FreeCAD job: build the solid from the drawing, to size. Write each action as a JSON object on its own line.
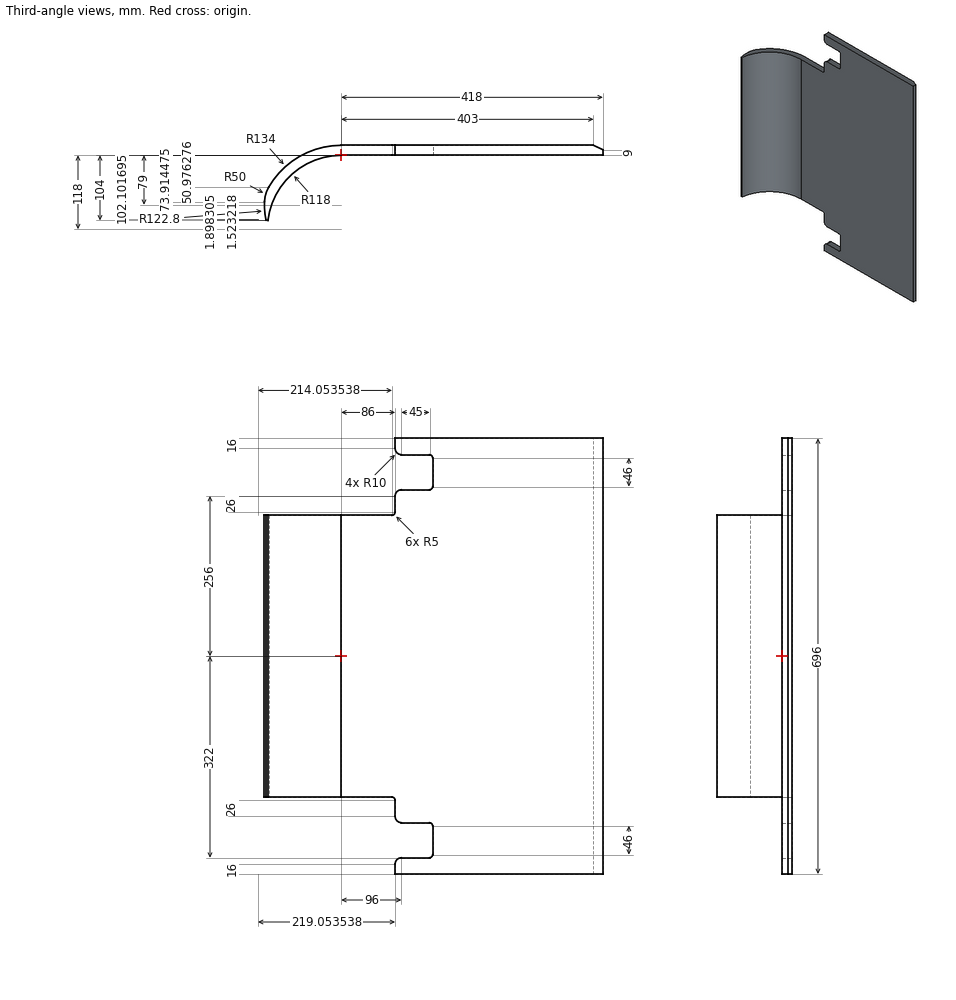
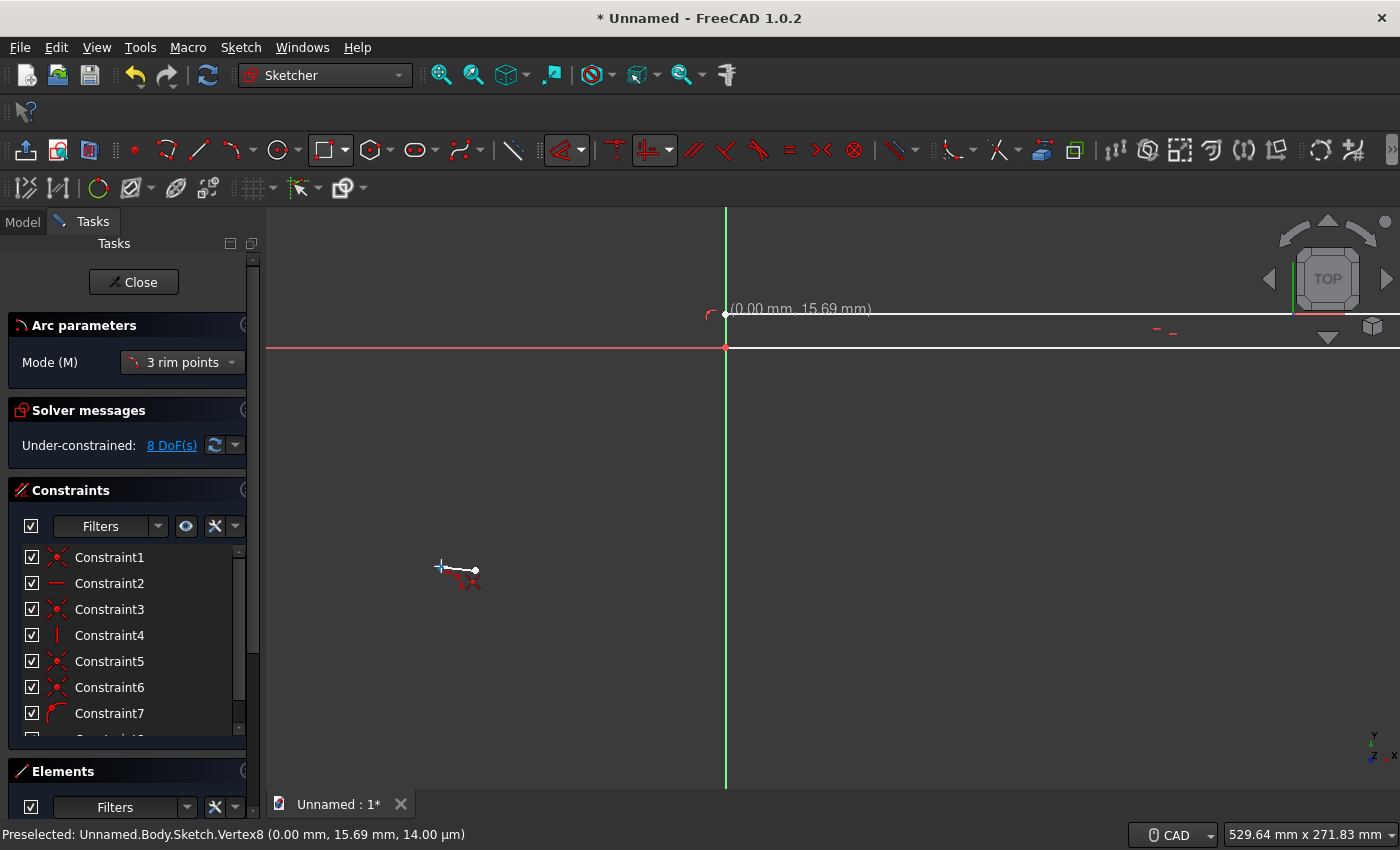
{"action": "left_click", "coordinate": [441, 567]}
{"action": "left_click", "coordinate": [535, 386]}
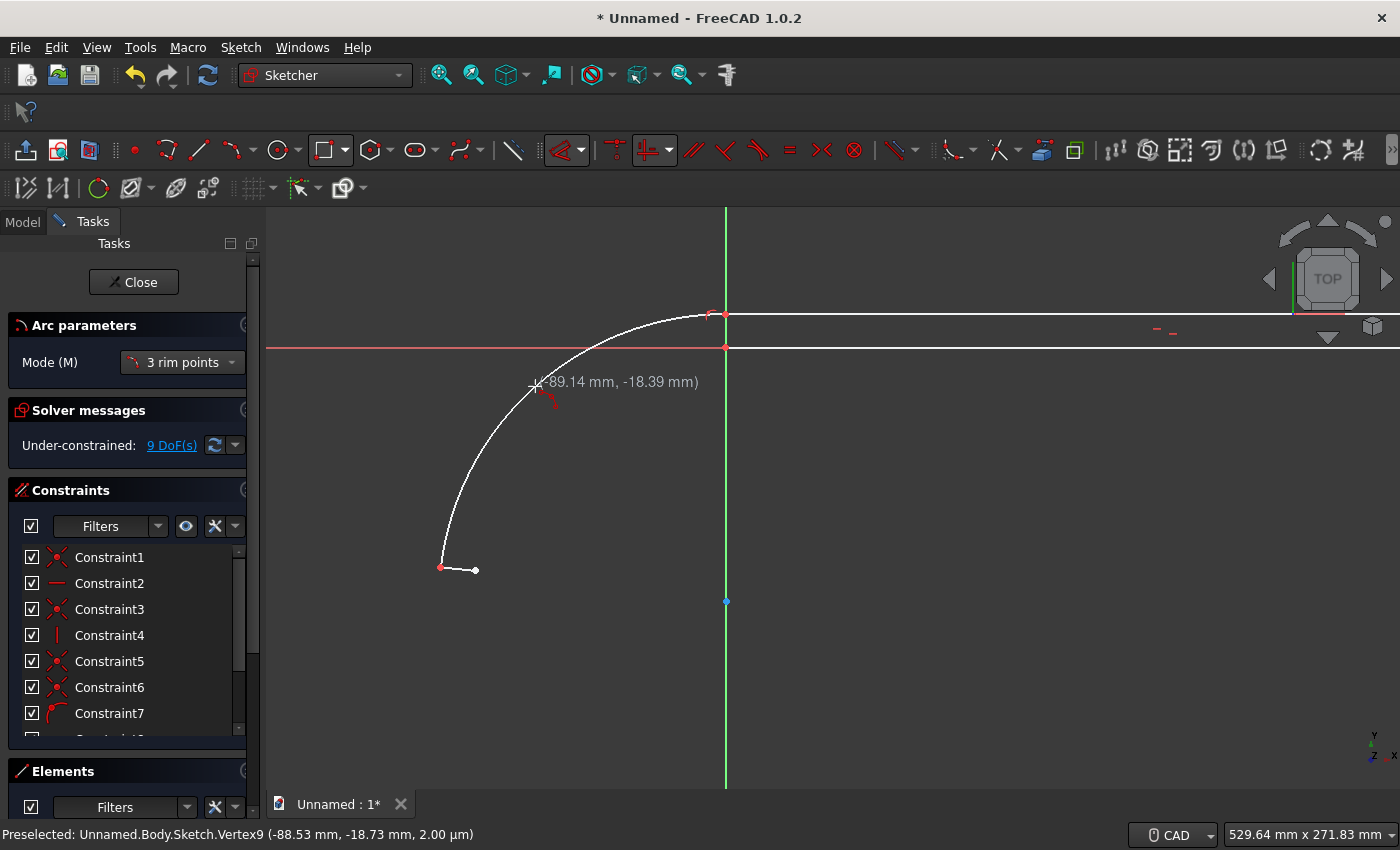
{"action": "left_click", "coordinate": [475, 571]}
{"action": "left_click", "coordinate": [726, 348]}
{"action": "left_click", "coordinate": [558, 411]}
{"action": "key", "text": "Escape"}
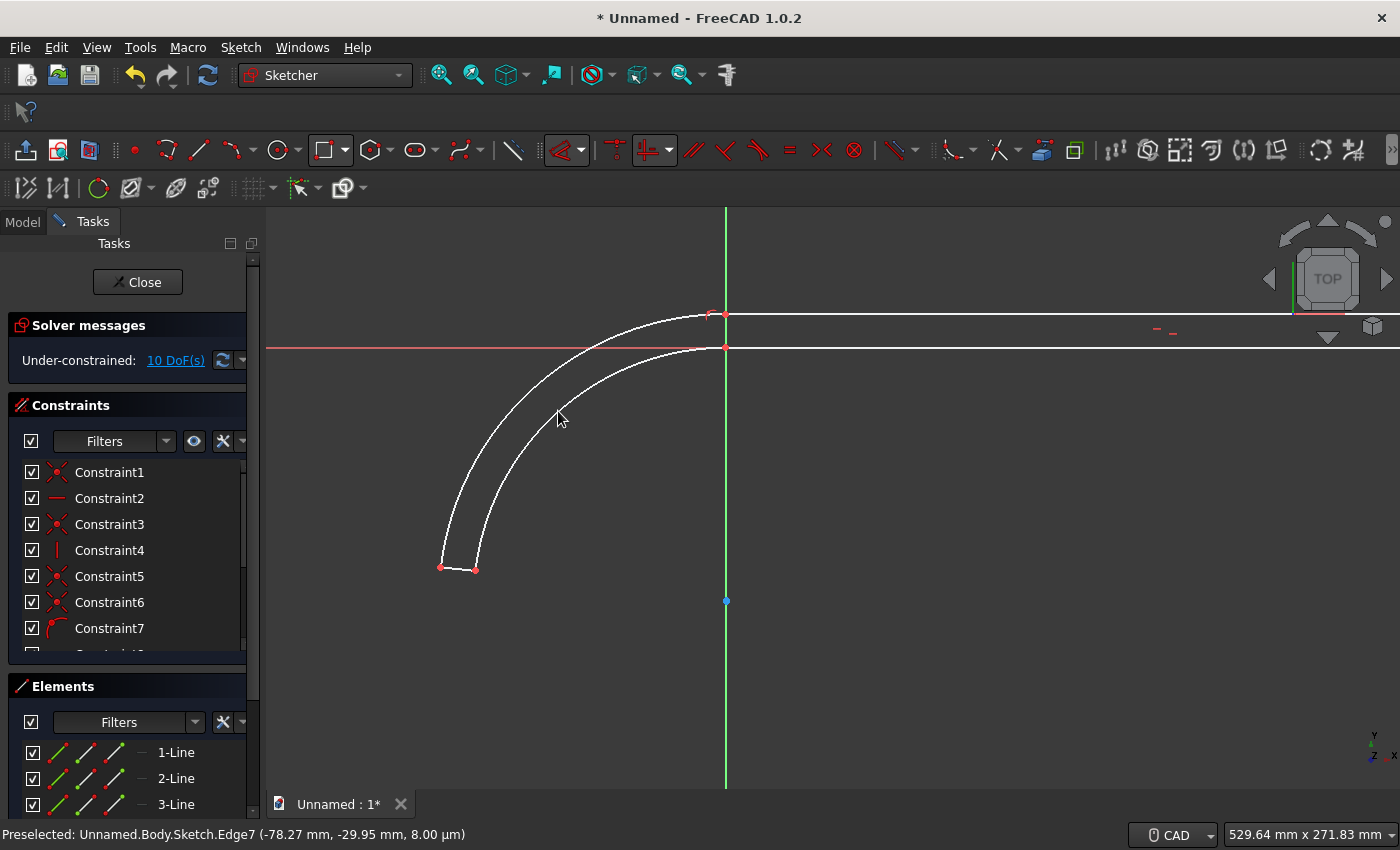
{"action": "left_click", "coordinate": [482, 450]}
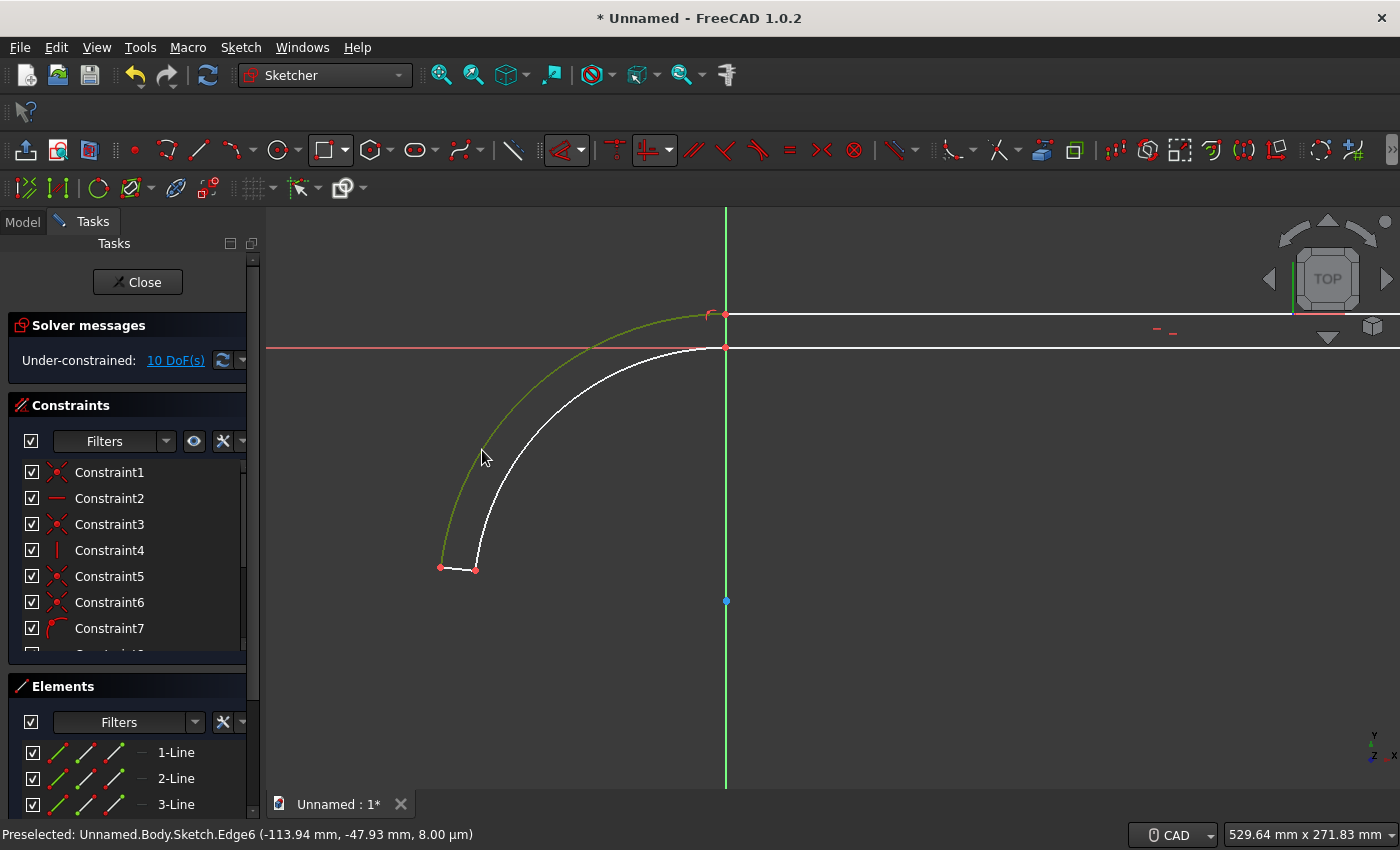
{"action": "left_click", "coordinate": [619, 371]}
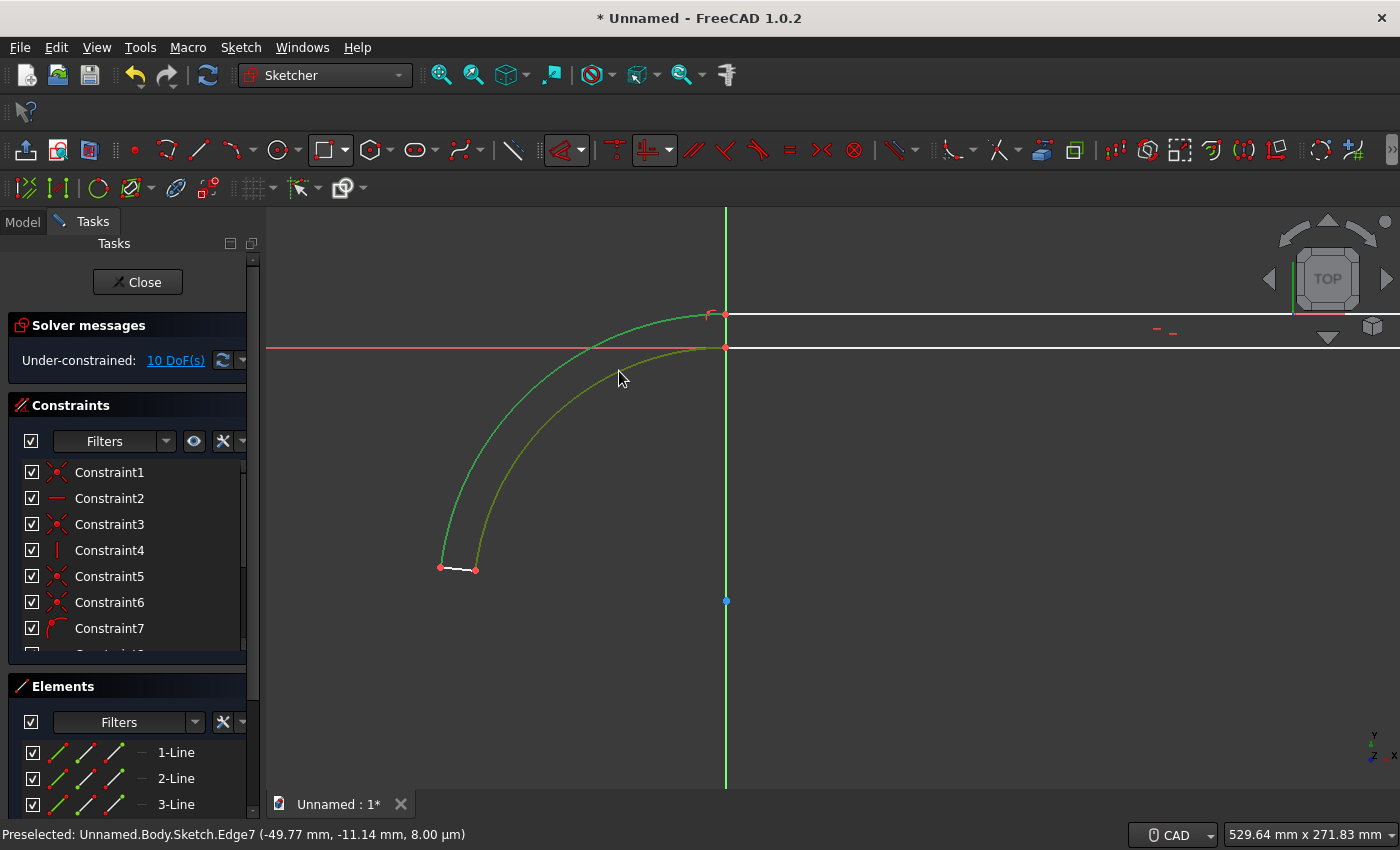
{"action": "left_click", "coordinate": [616, 150]}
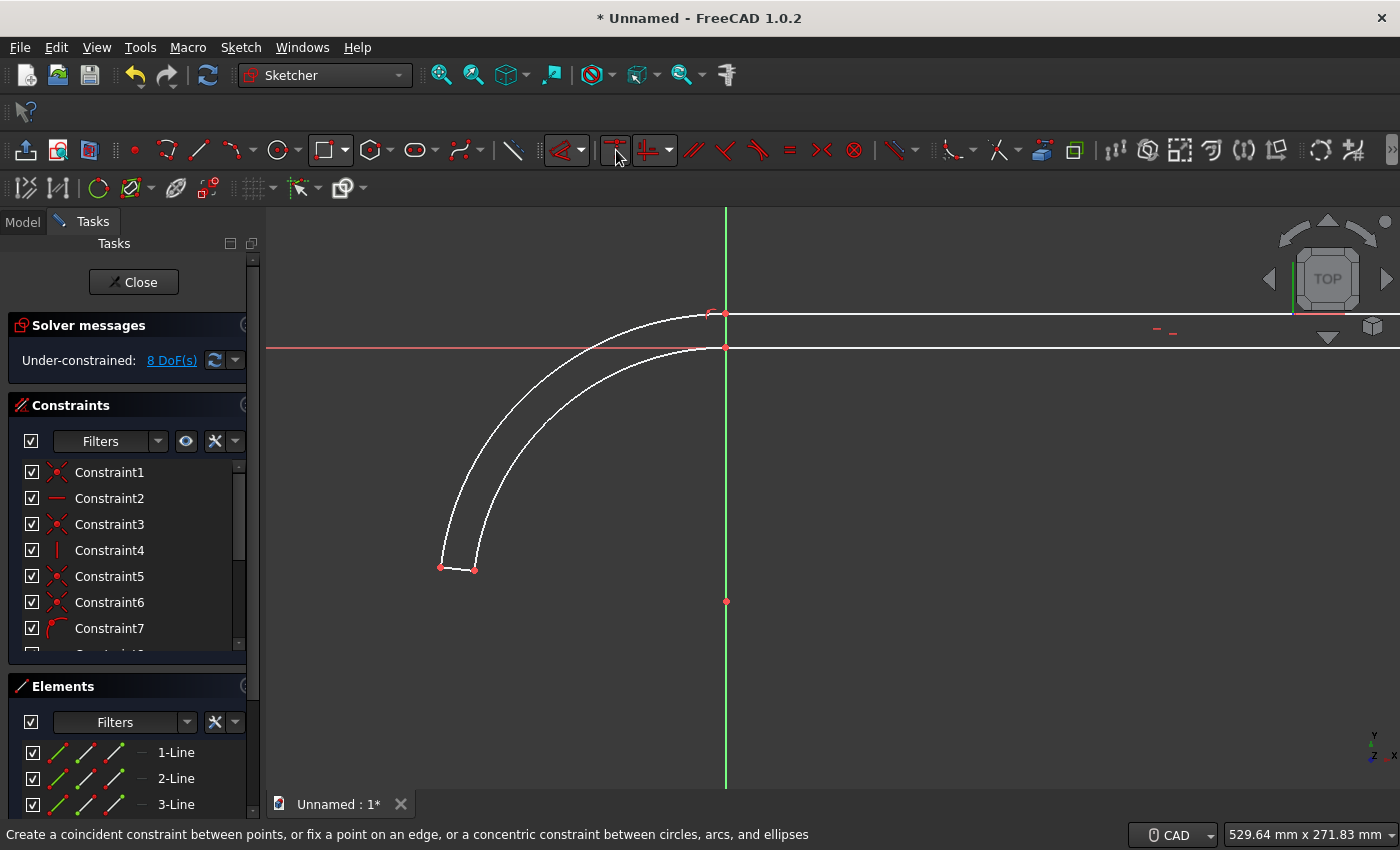
{"action": "left_click", "coordinate": [727, 602]}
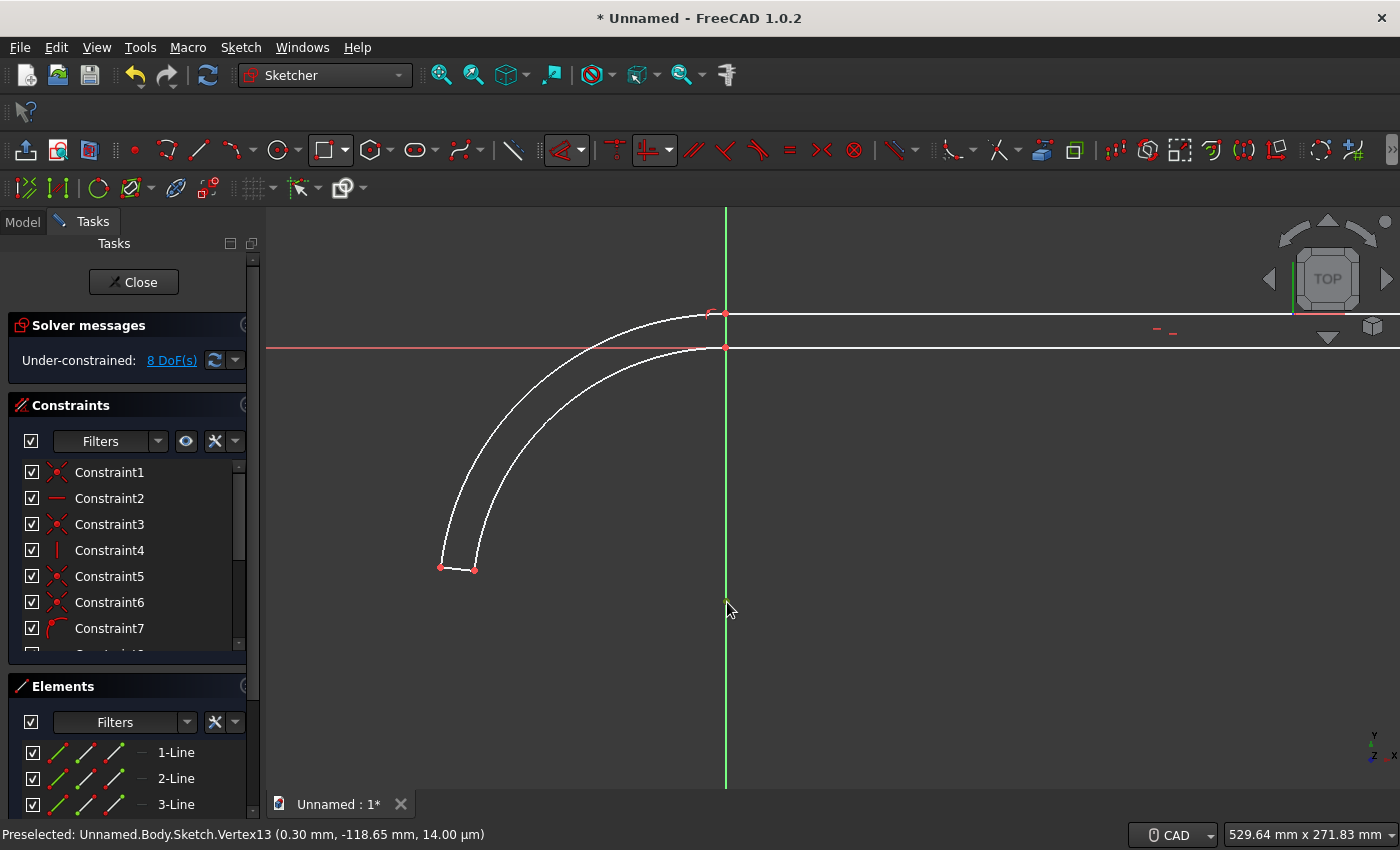
{"action": "left_click", "coordinate": [726, 723]}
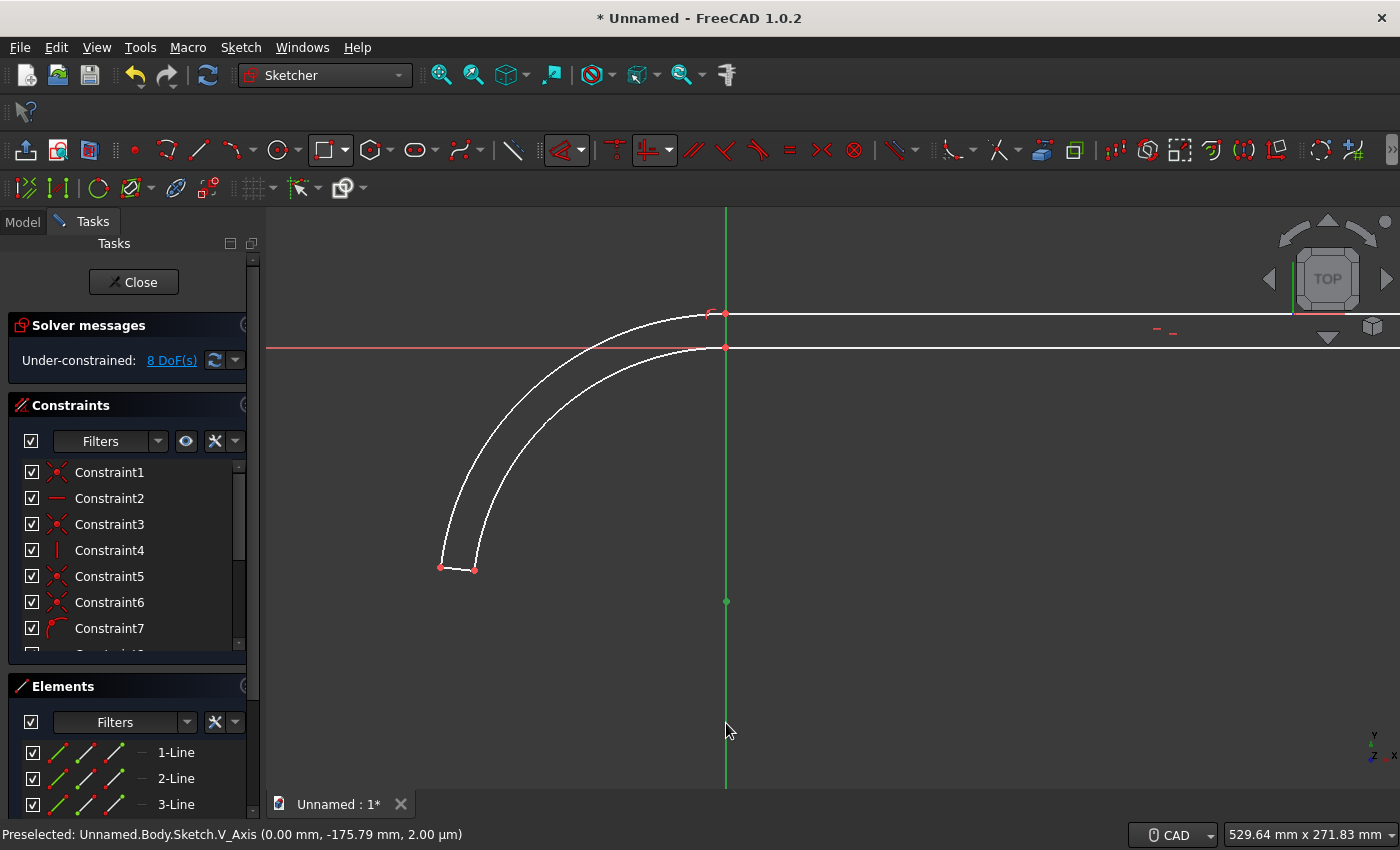
{"action": "left_click", "coordinate": [616, 150]}